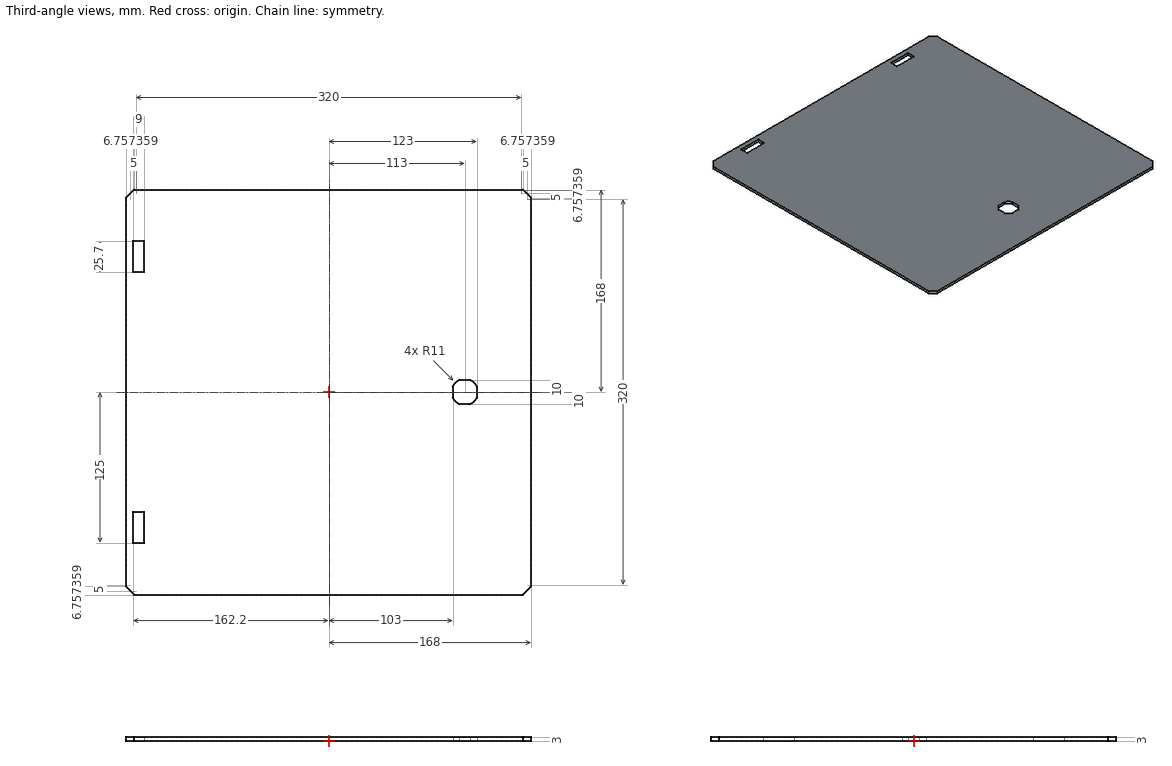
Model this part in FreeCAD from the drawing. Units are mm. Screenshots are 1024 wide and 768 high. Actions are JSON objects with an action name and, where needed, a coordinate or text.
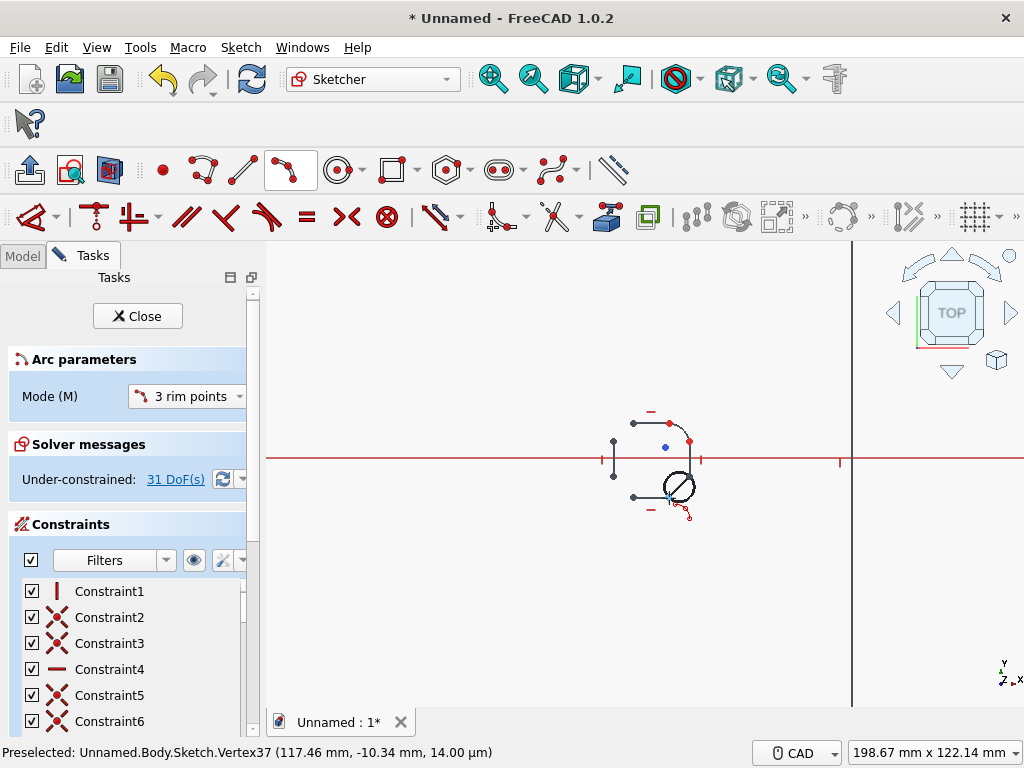
{"action": "scroll", "coordinate": [682, 488], "scroll_direction": "up", "scroll_amount": 9}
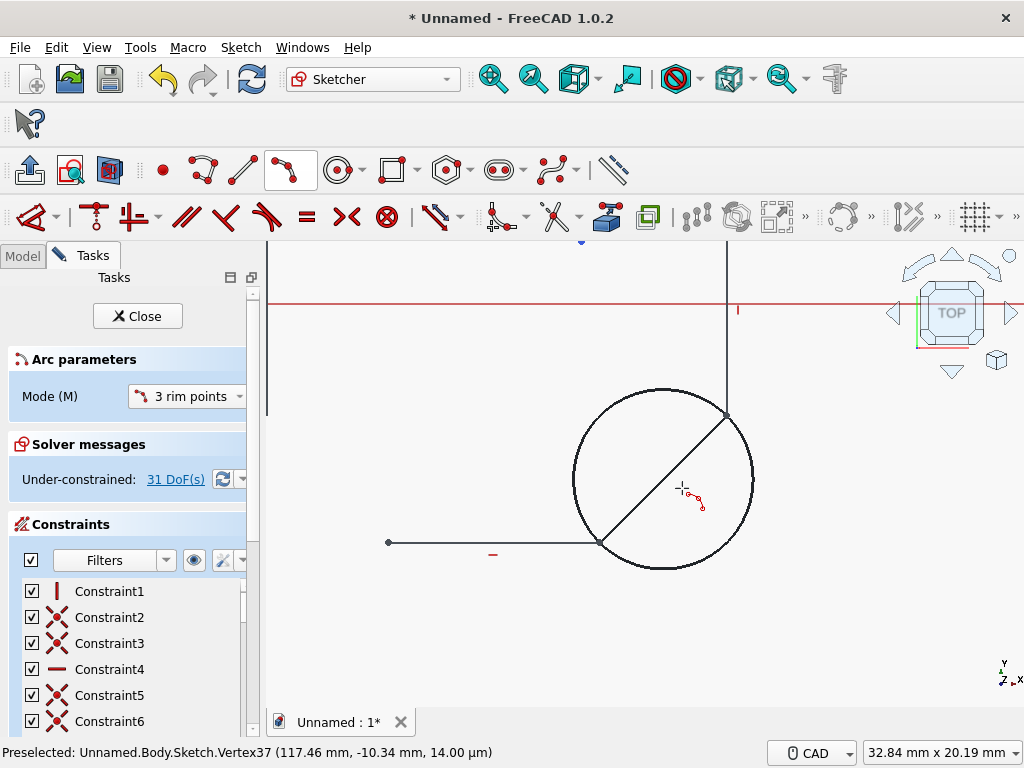
{"action": "left_click", "coordinate": [676, 484]}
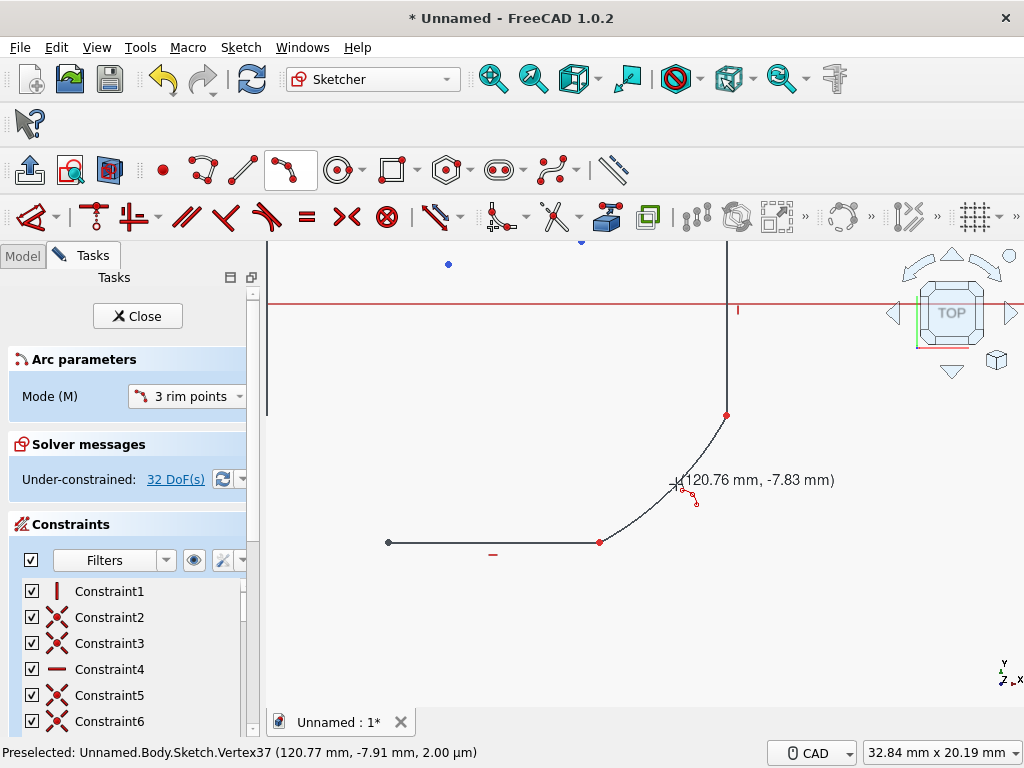
{"action": "scroll", "coordinate": [691, 481], "scroll_direction": "down", "scroll_amount": 16}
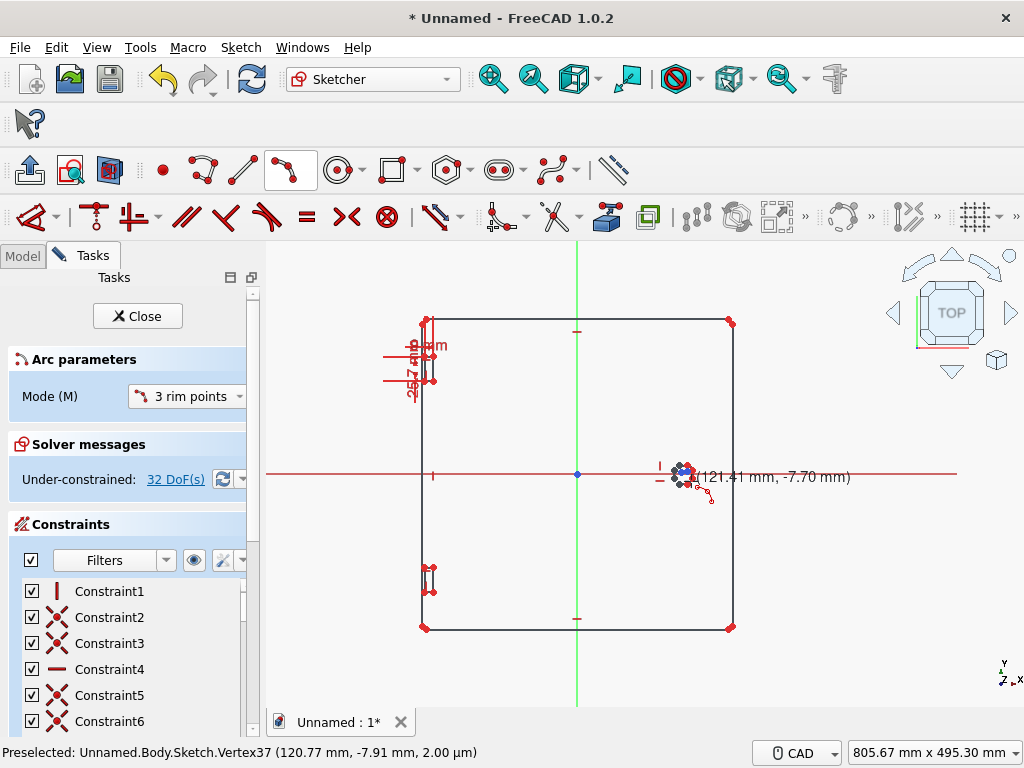
{"action": "scroll", "coordinate": [679, 484], "scroll_direction": "up", "scroll_amount": 7}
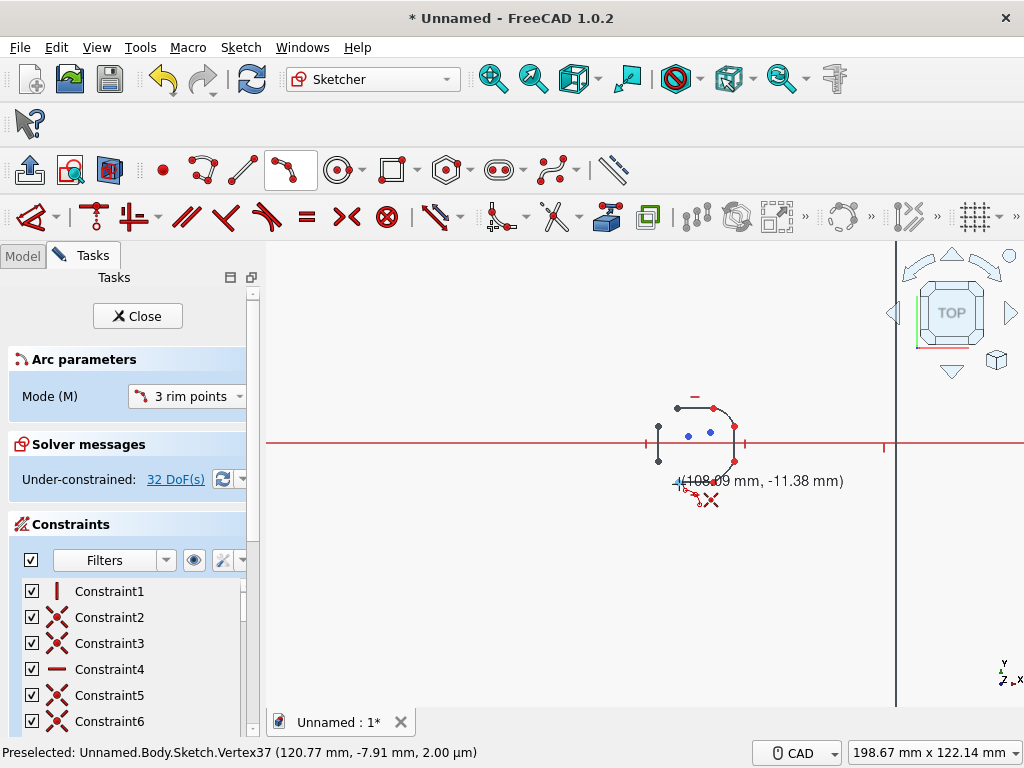
{"action": "left_click", "coordinate": [678, 482]}
{"action": "left_click", "coordinate": [658, 461]}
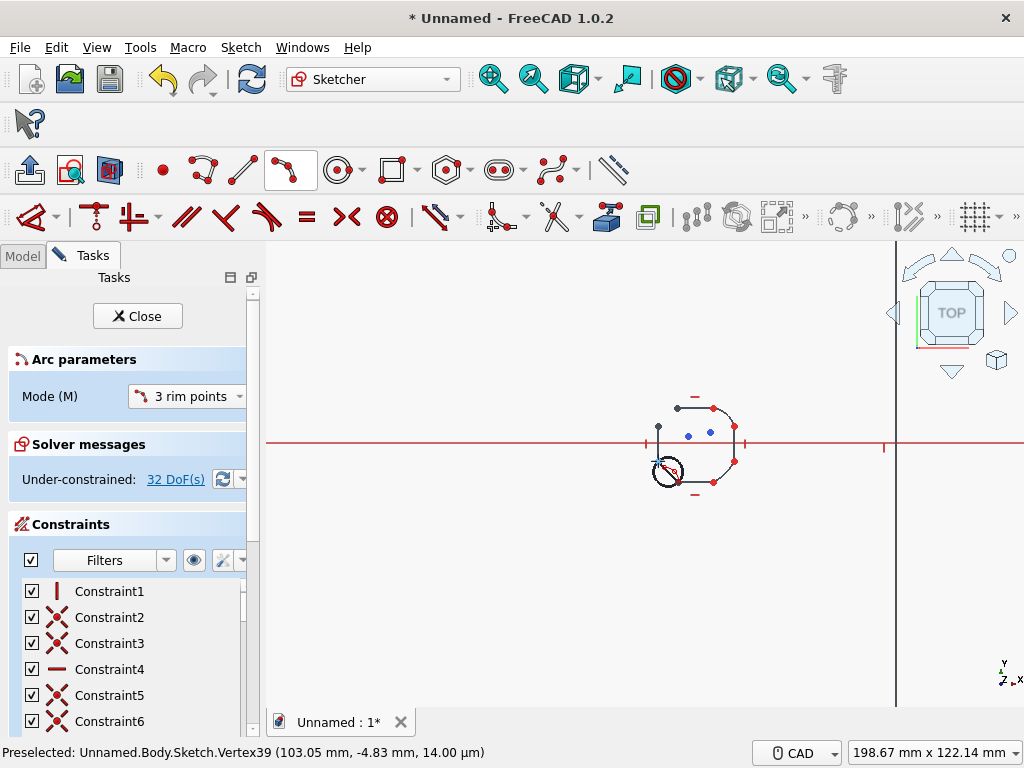
{"action": "scroll", "coordinate": [666, 473], "scroll_direction": "up", "scroll_amount": 9}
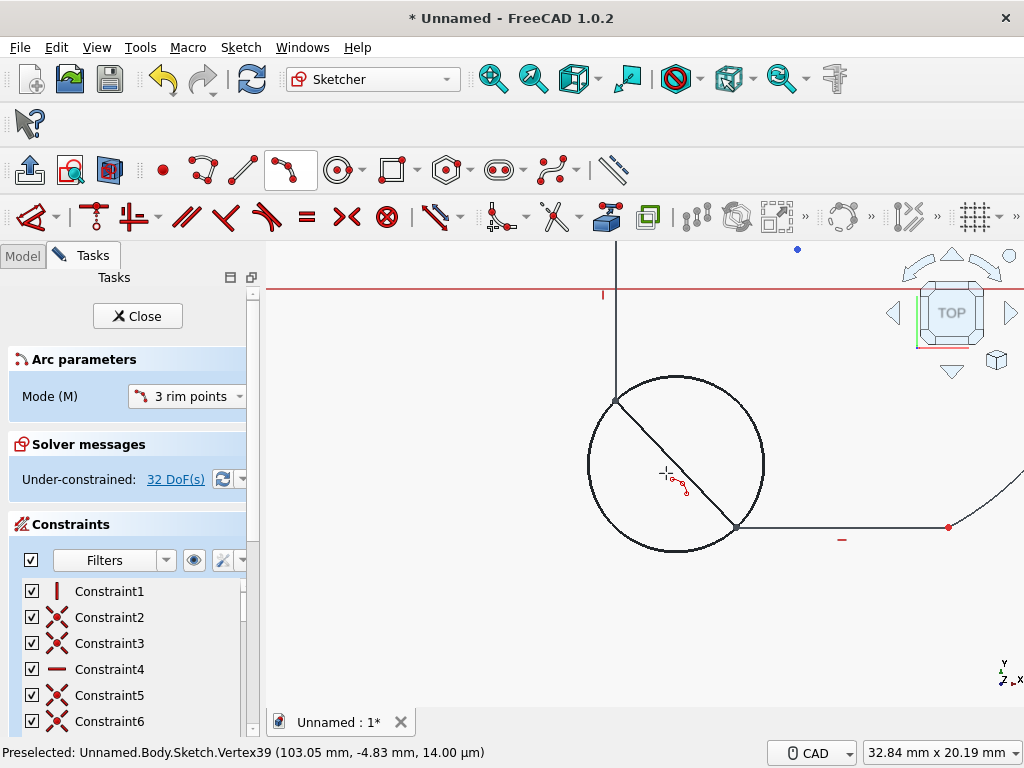
{"action": "left_click", "coordinate": [666, 469]}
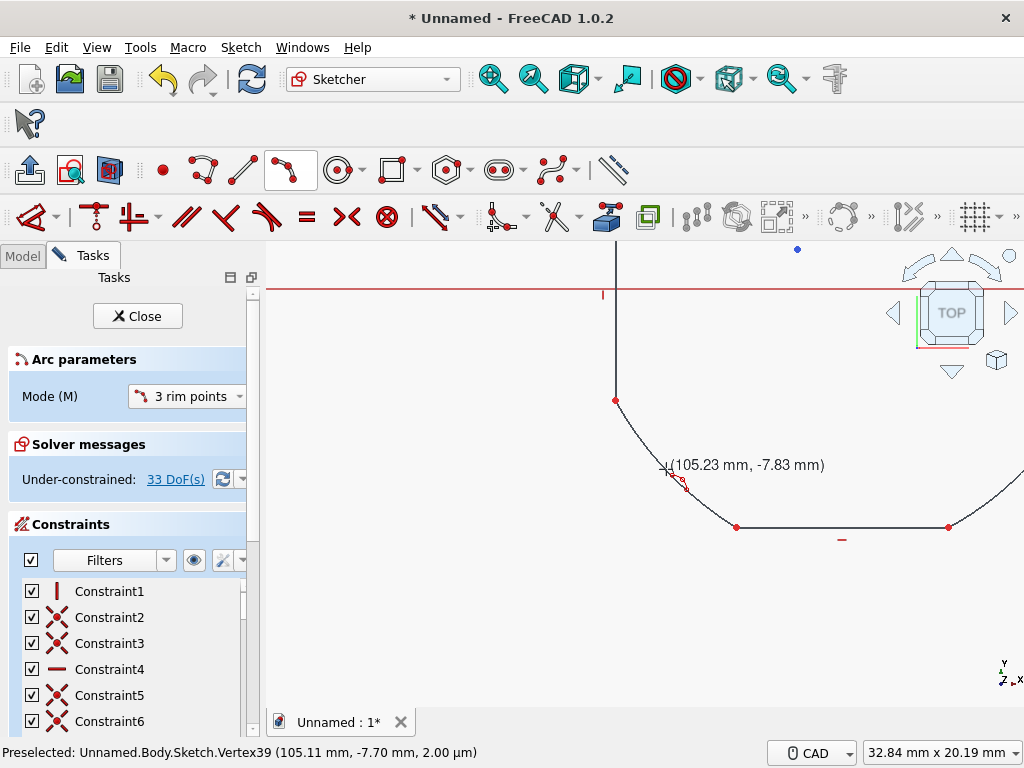
{"action": "scroll", "coordinate": [676, 482], "scroll_direction": "down", "scroll_amount": 16}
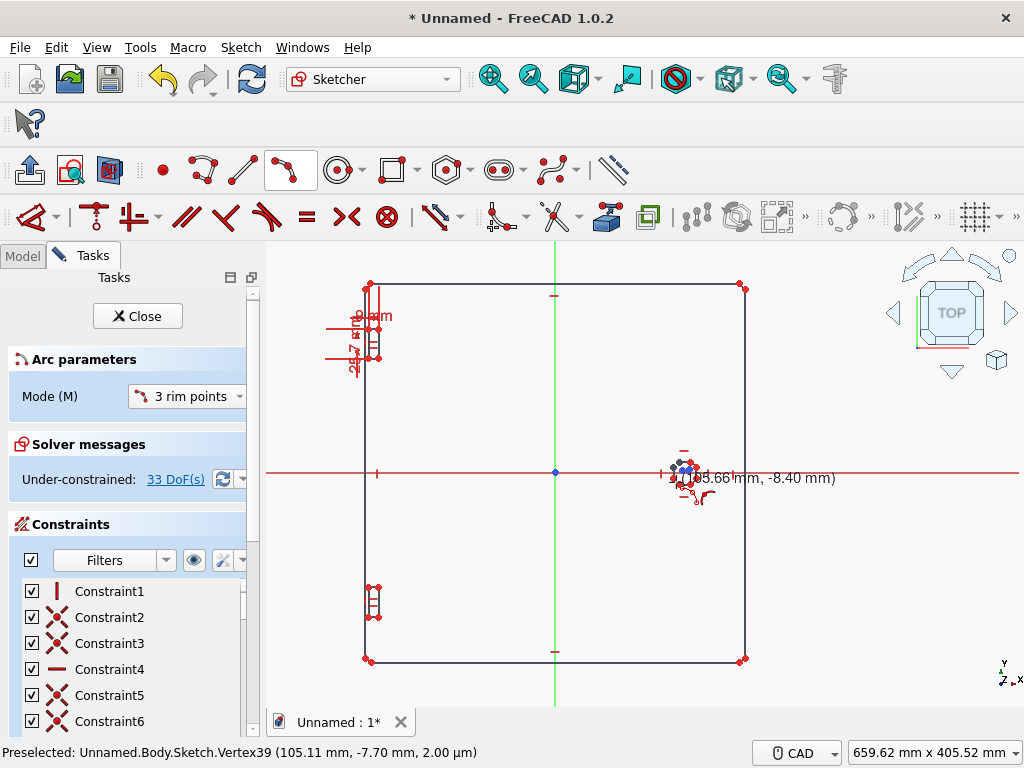
{"action": "scroll", "coordinate": [674, 470], "scroll_direction": "up", "scroll_amount": 7}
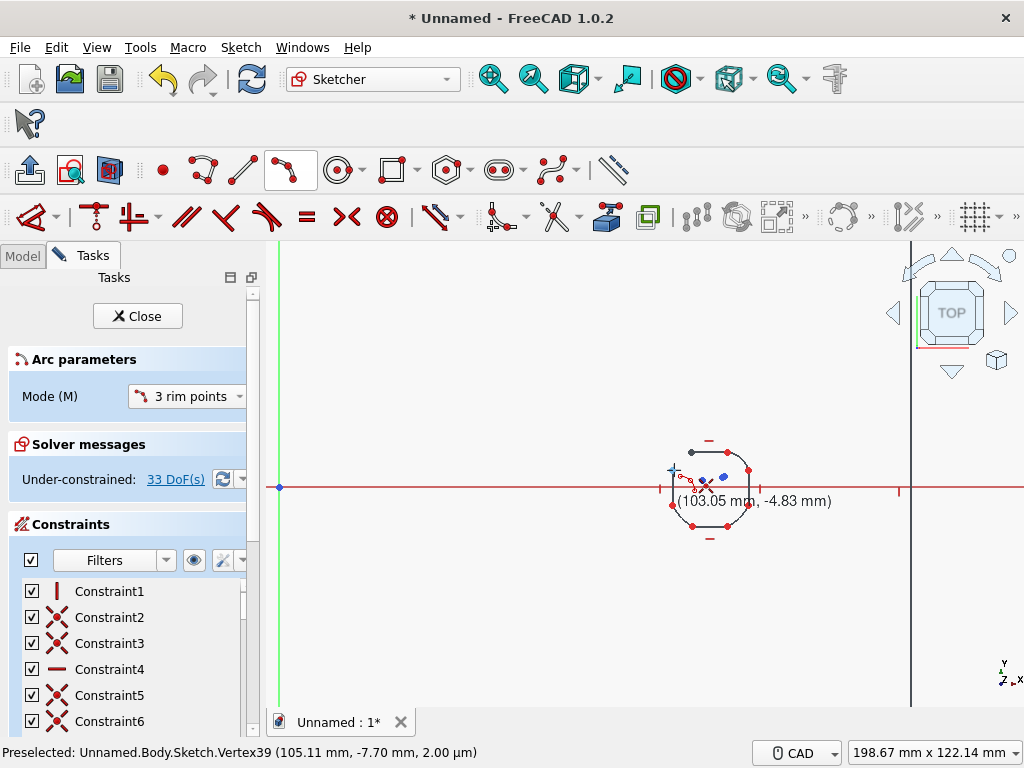
{"action": "left_click", "coordinate": [673, 471]}
{"action": "left_click", "coordinate": [692, 452]}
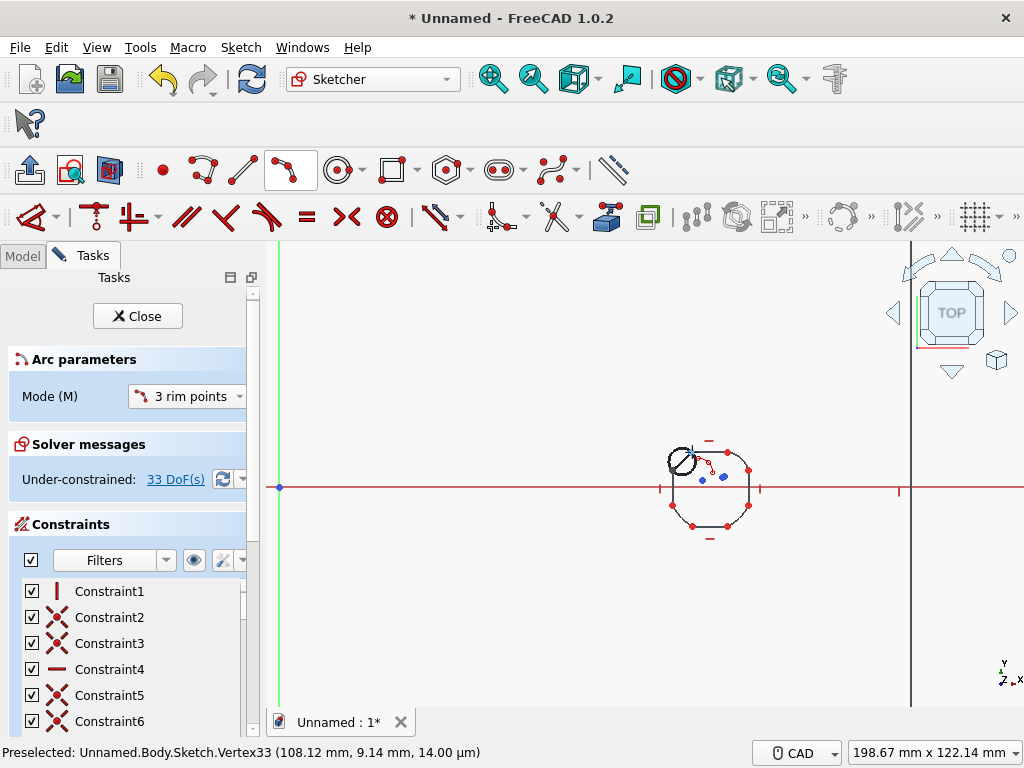
{"action": "scroll", "coordinate": [681, 458], "scroll_direction": "up", "scroll_amount": 9}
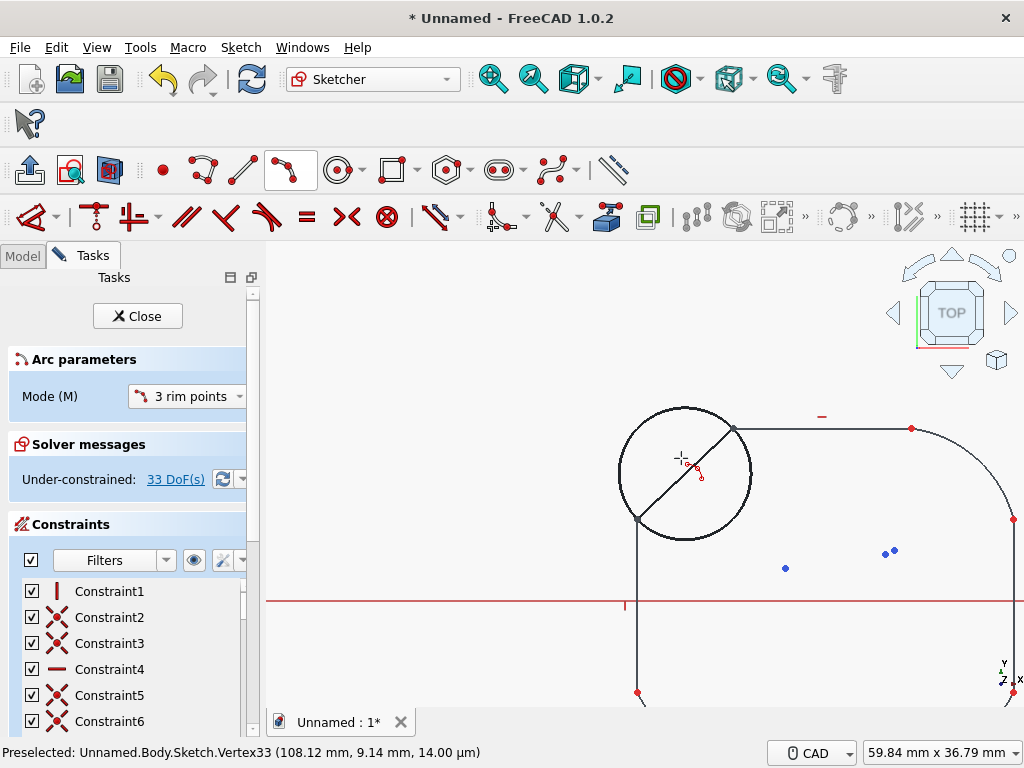
{"action": "left_click", "coordinate": [678, 453]}
{"action": "key", "text": "Escape"}